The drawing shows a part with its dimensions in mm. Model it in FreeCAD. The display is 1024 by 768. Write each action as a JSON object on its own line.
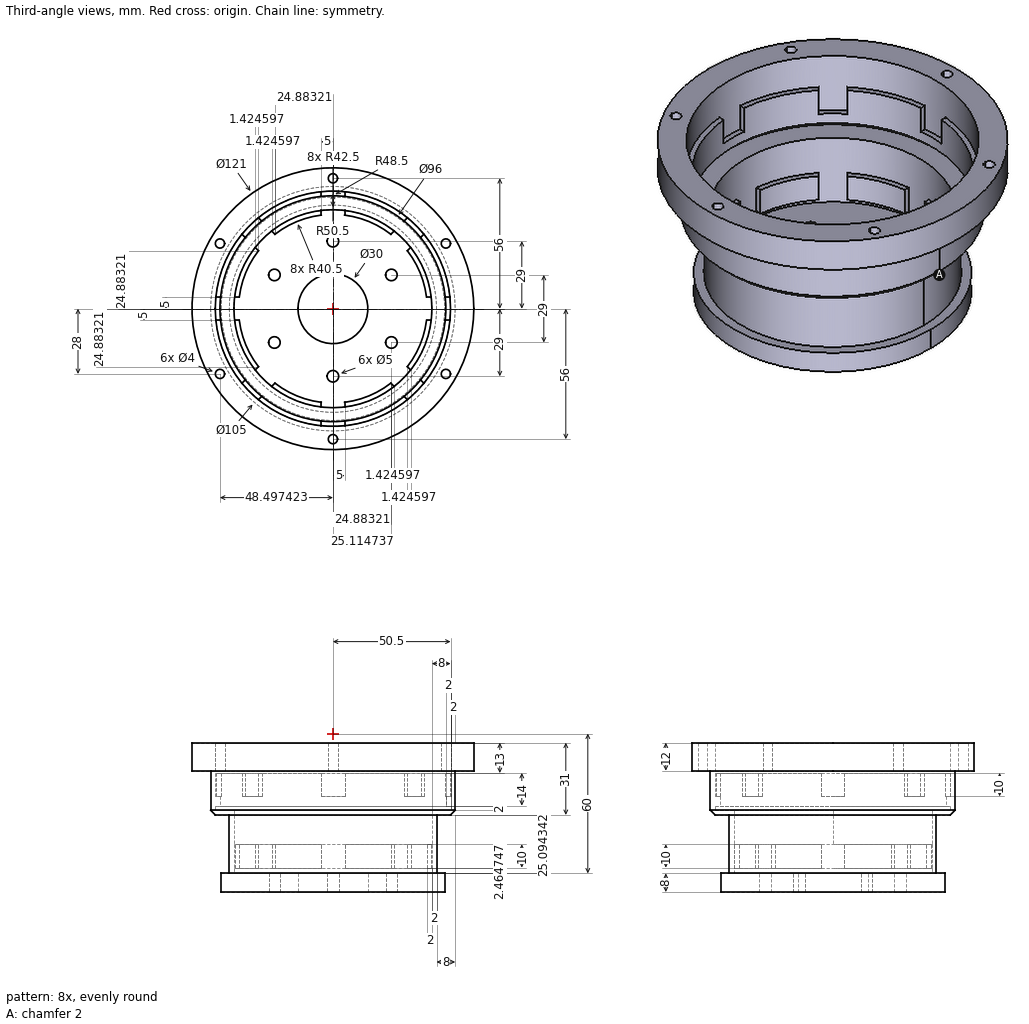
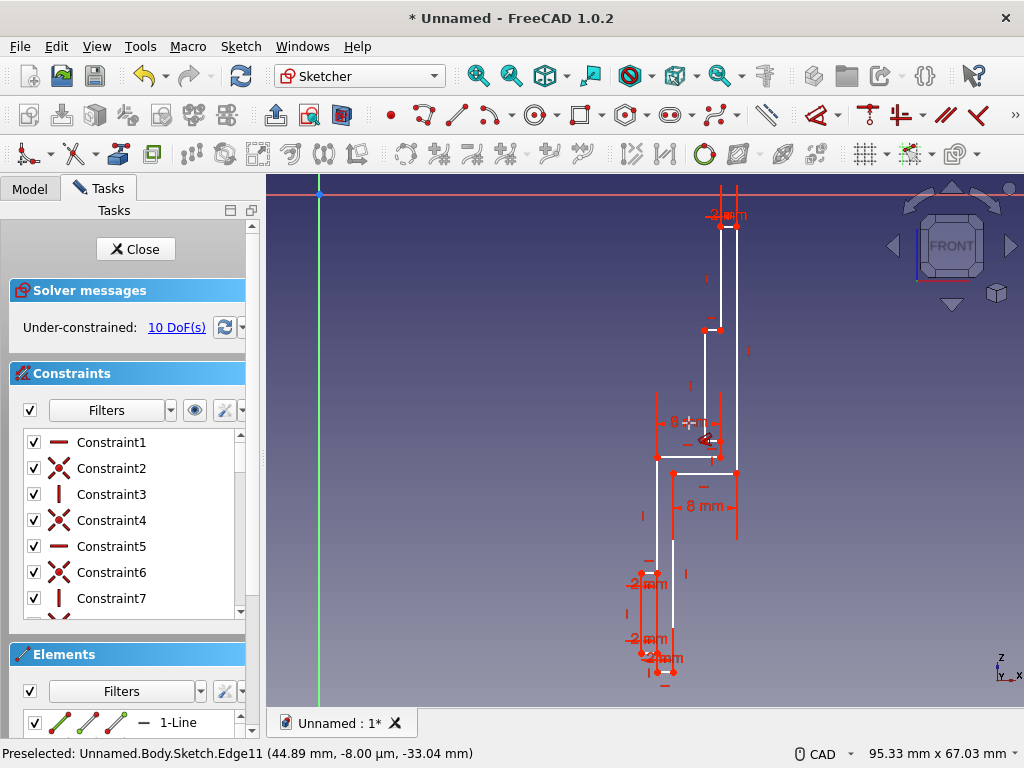
{"action": "scroll", "coordinate": [721, 449], "scroll_direction": "up", "scroll_amount": 5}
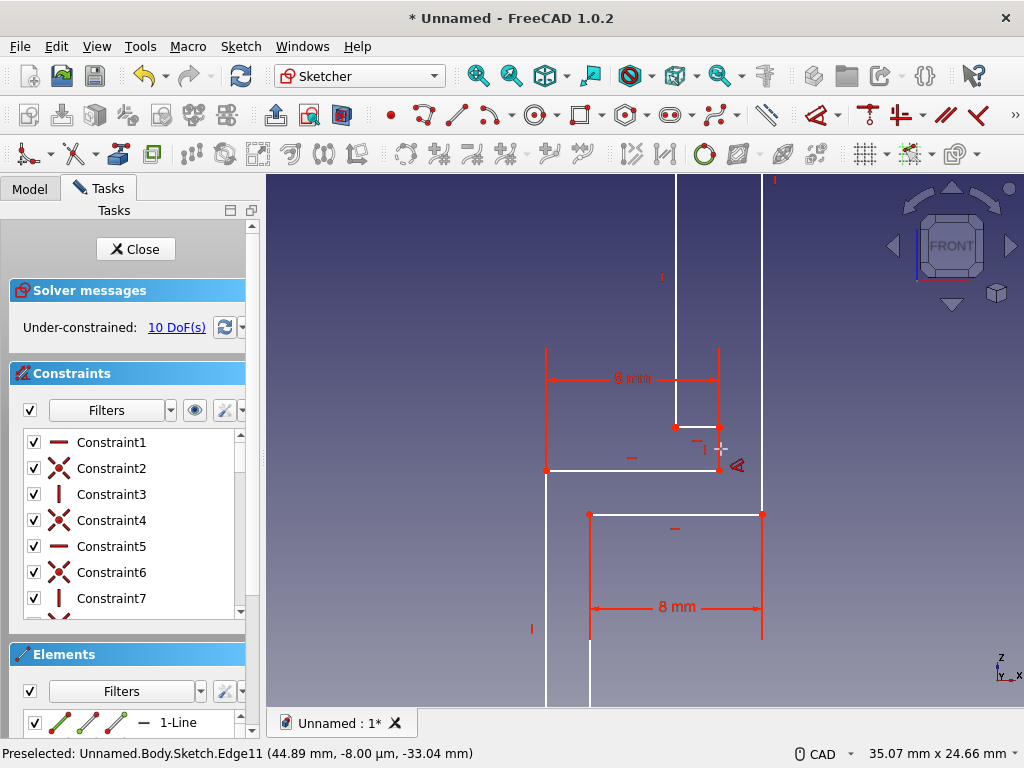
{"action": "left_click", "coordinate": [719, 449]}
{"action": "left_click", "coordinate": [685, 449]}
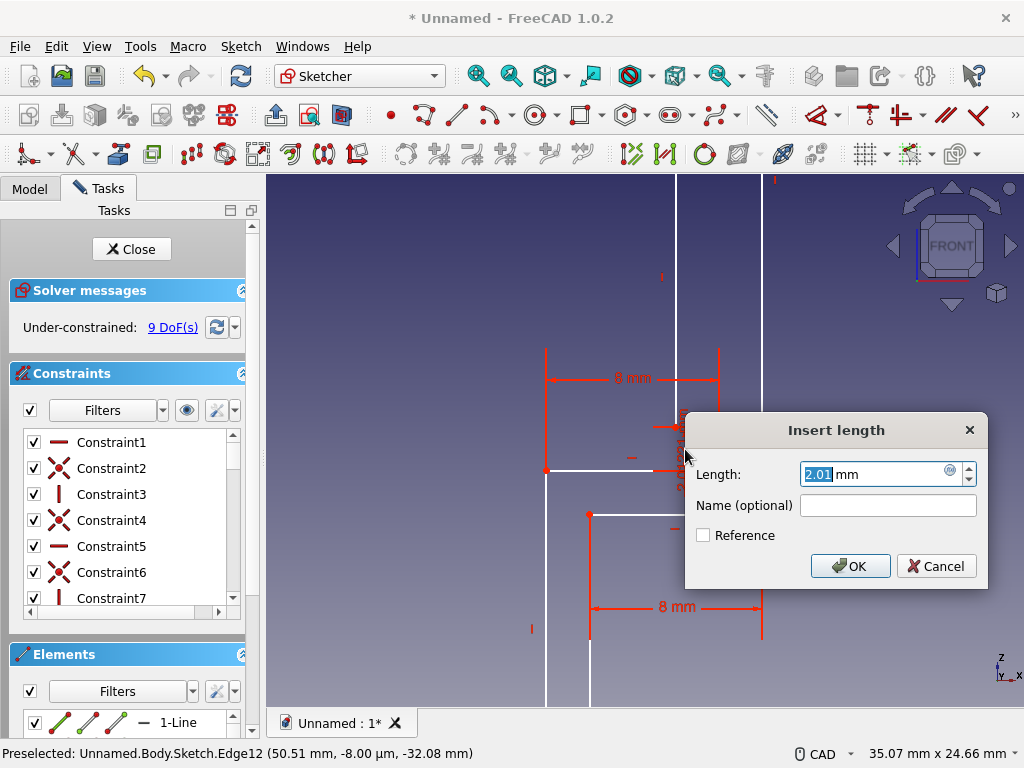
{"action": "type", "text": "2"}
{"action": "key", "text": "Return"}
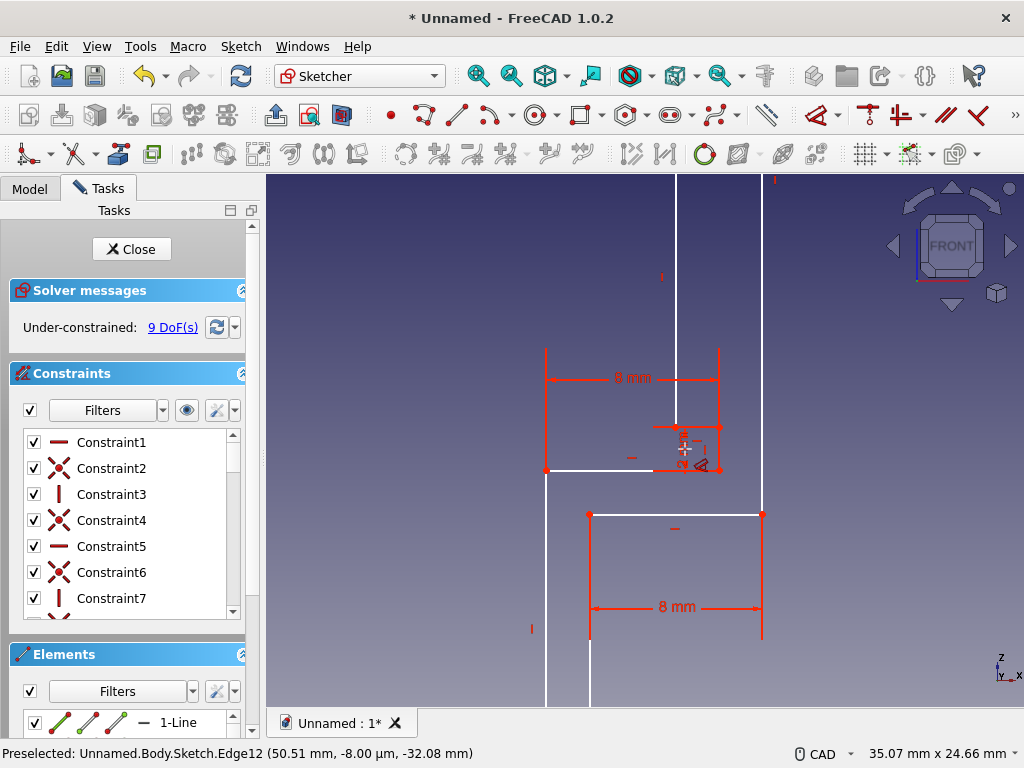
{"action": "left_click", "coordinate": [706, 427]}
{"action": "left_click", "coordinate": [707, 393]}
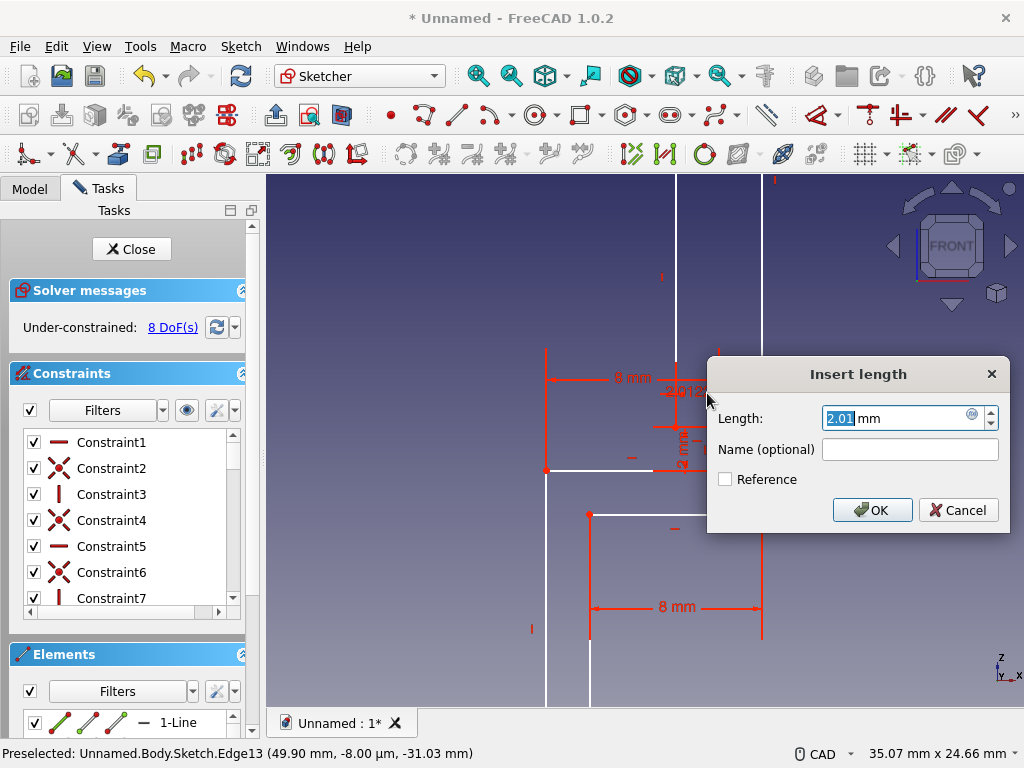
{"action": "type", "text": "2"}
{"action": "key", "text": "Return"}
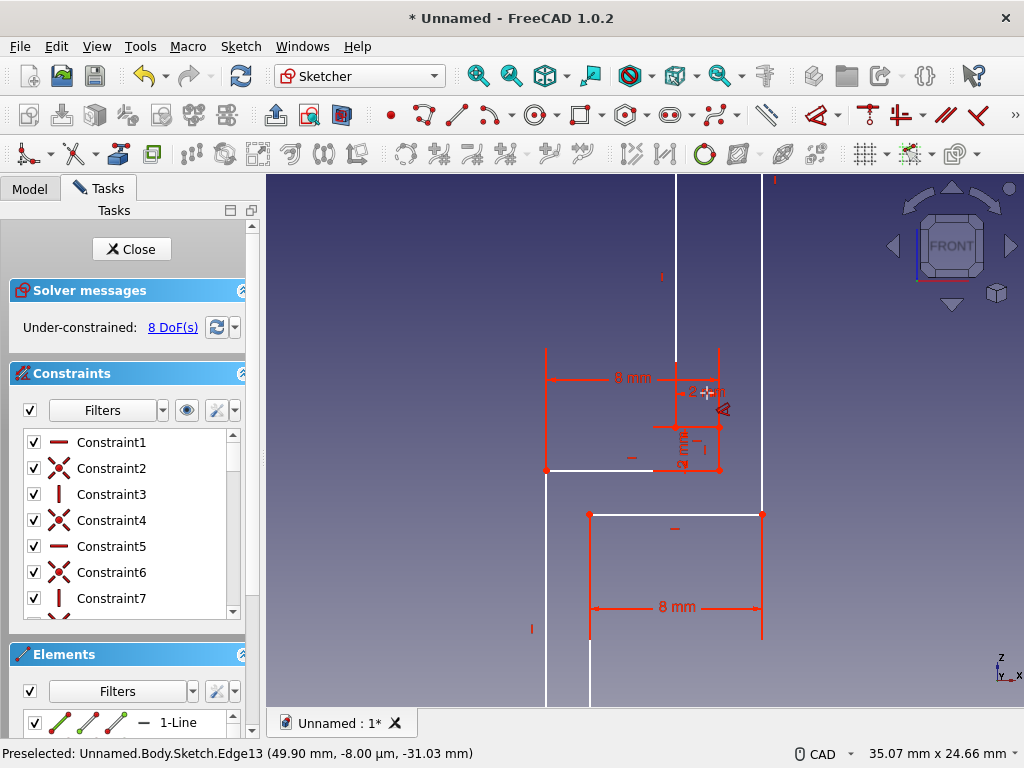
{"action": "scroll", "coordinate": [701, 452], "scroll_direction": "down", "scroll_amount": 7}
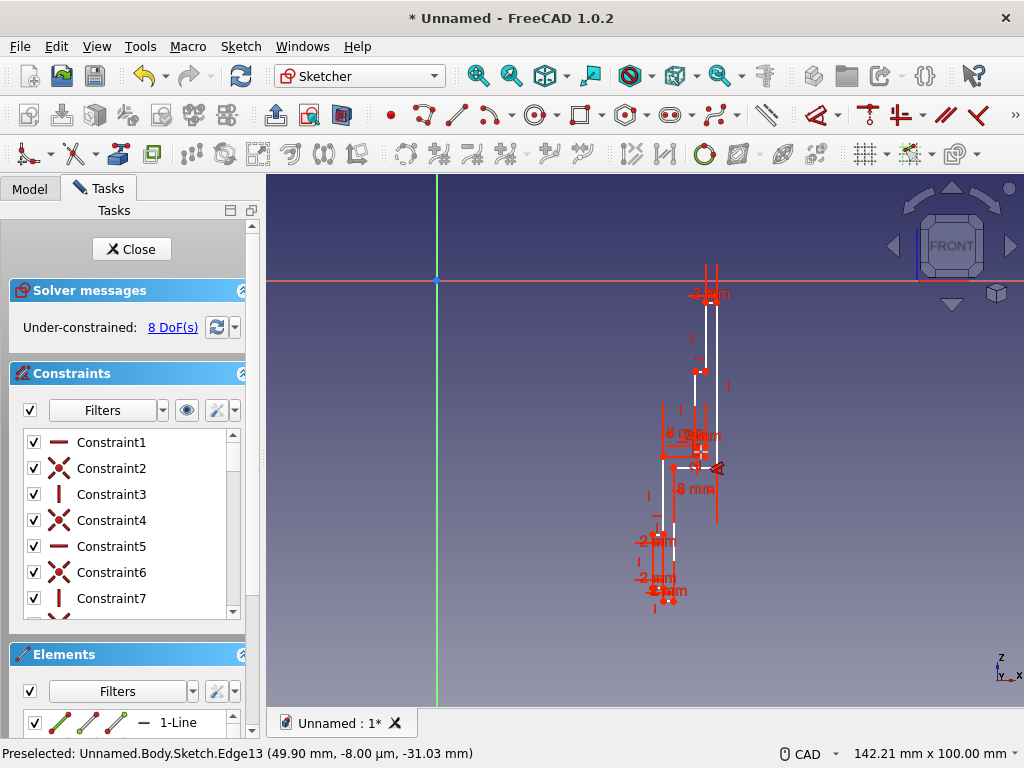
{"action": "left_click", "coordinate": [717, 418]}
{"action": "left_click", "coordinate": [751, 385]}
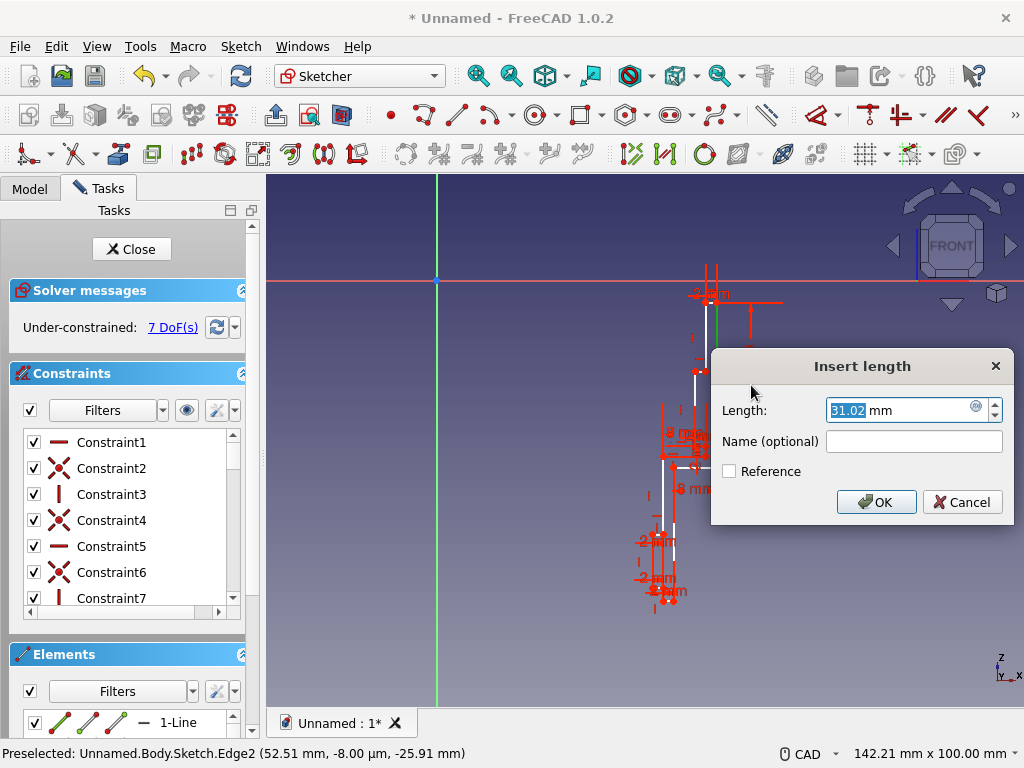
{"action": "type", "text": "31"}
{"action": "key", "text": "Return"}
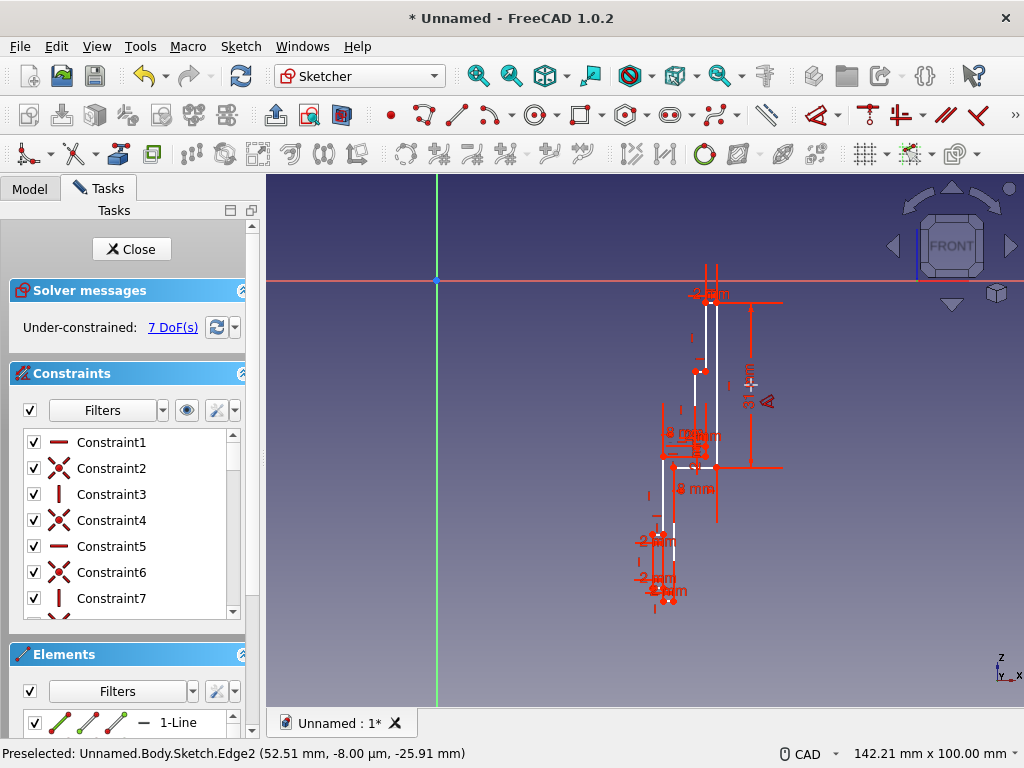
{"action": "left_click", "coordinate": [653, 572]}
{"action": "left_click", "coordinate": [735, 562]}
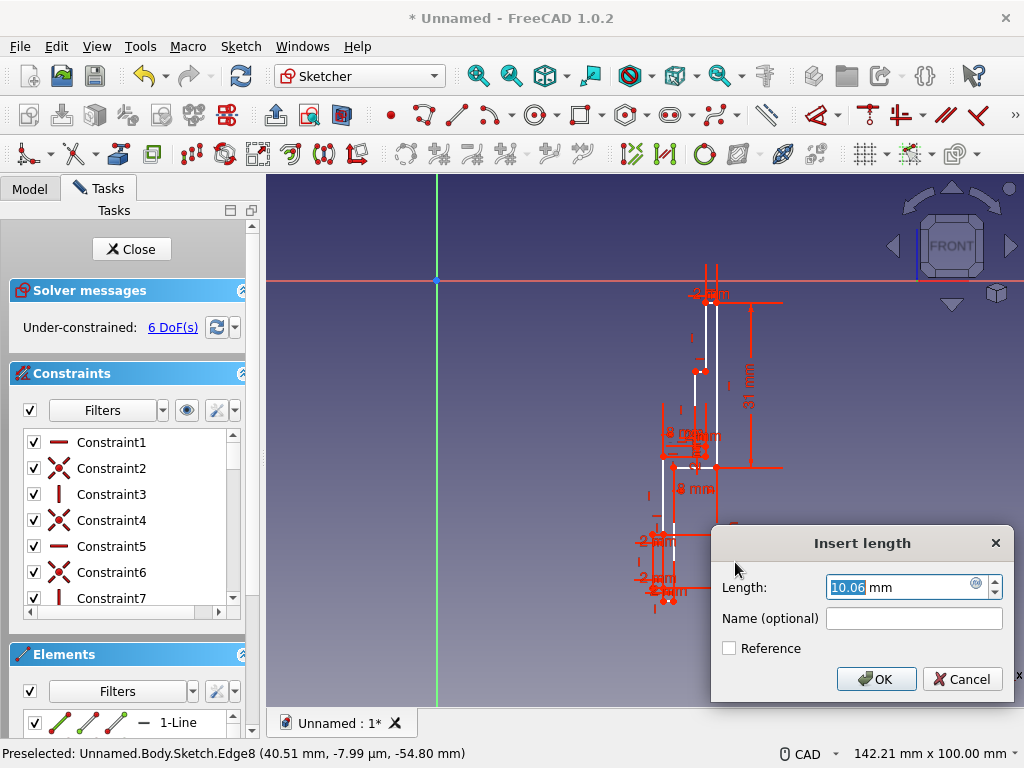
{"action": "type", "text": "10"}
{"action": "key", "text": "Return"}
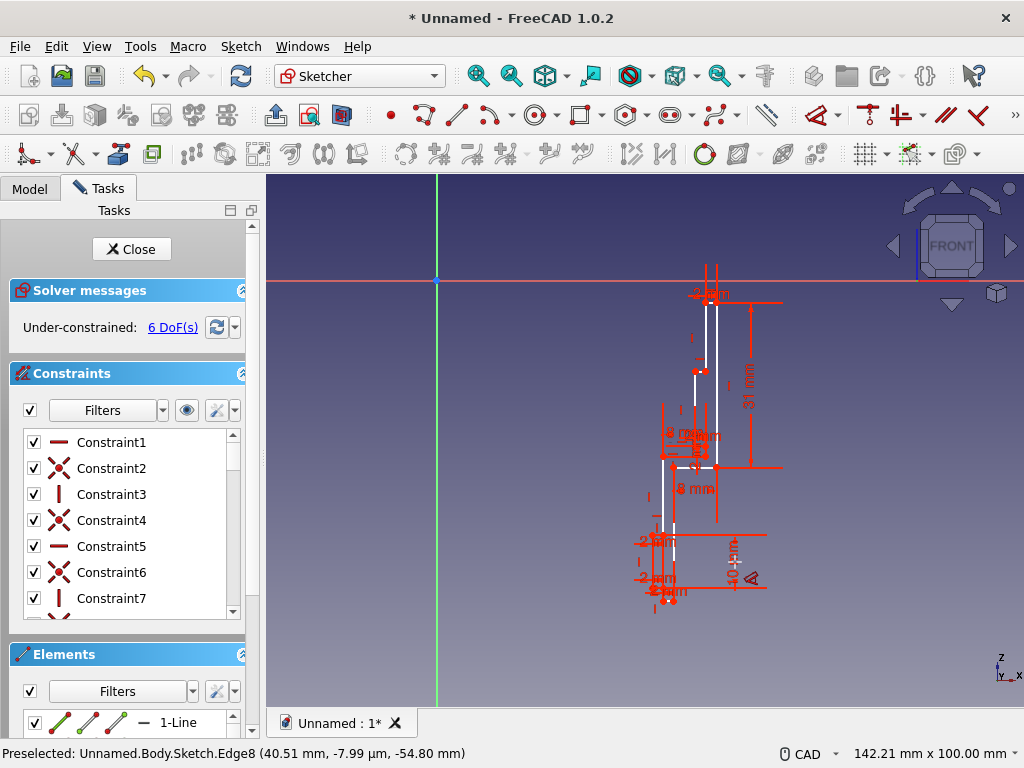
{"action": "left_click", "coordinate": [695, 424]}
{"action": "left_click", "coordinate": [661, 409]}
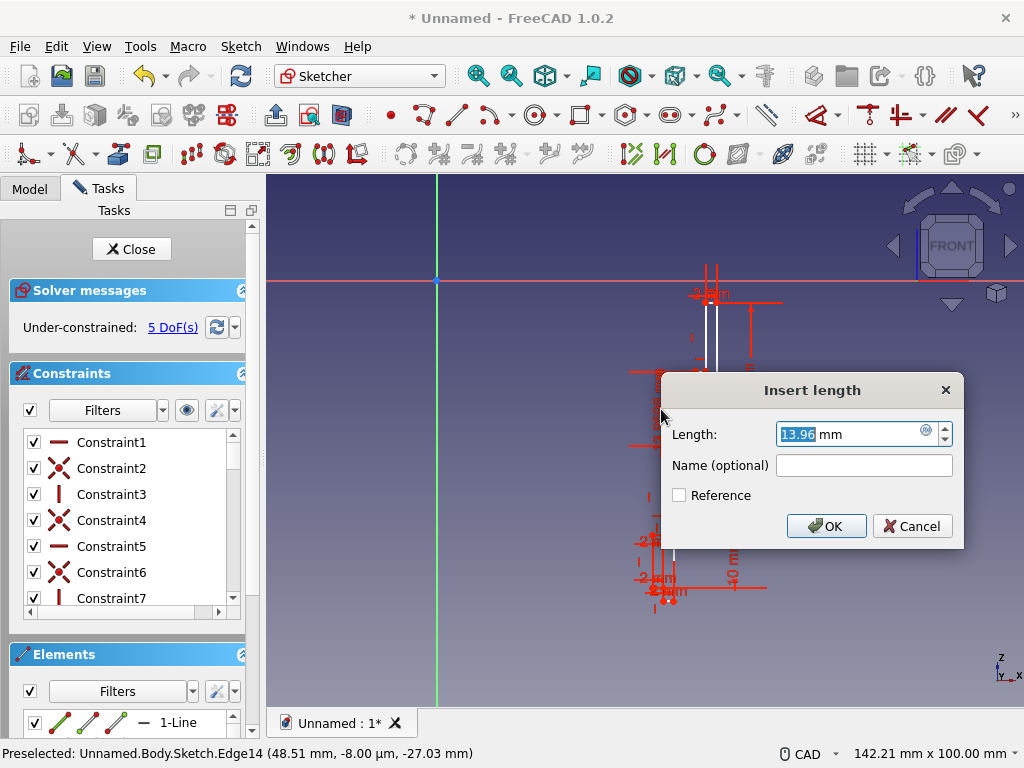
{"action": "type", "text": "14"}
{"action": "key", "text": "Return"}